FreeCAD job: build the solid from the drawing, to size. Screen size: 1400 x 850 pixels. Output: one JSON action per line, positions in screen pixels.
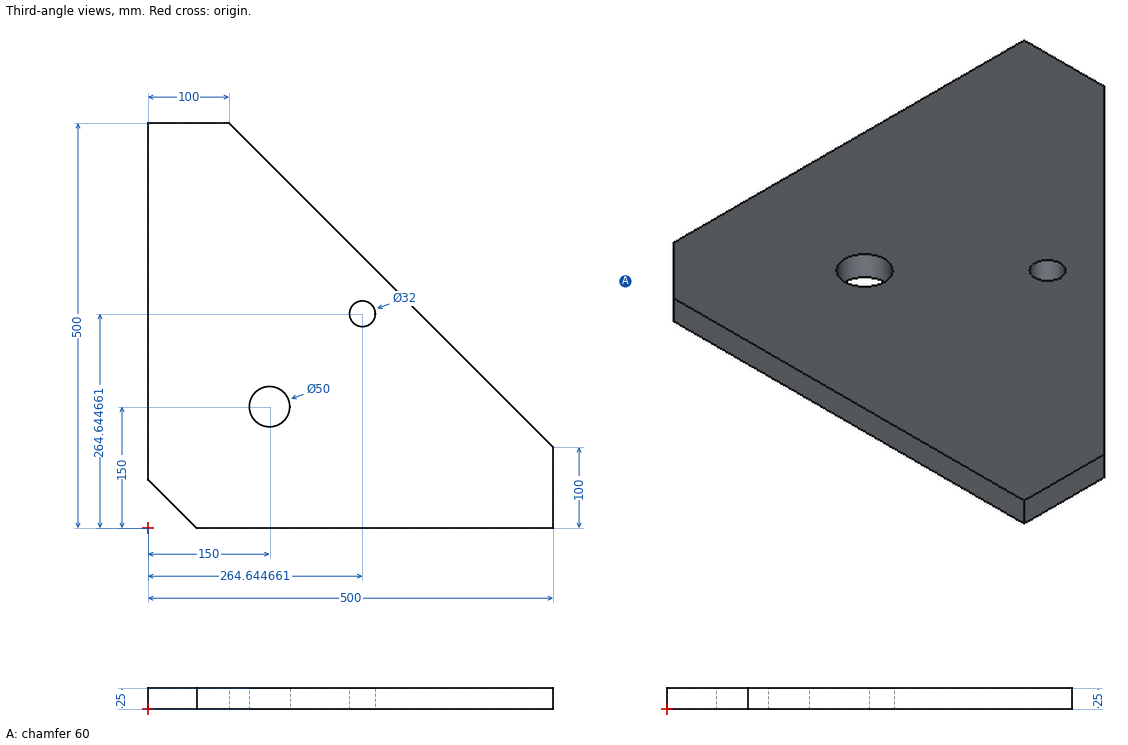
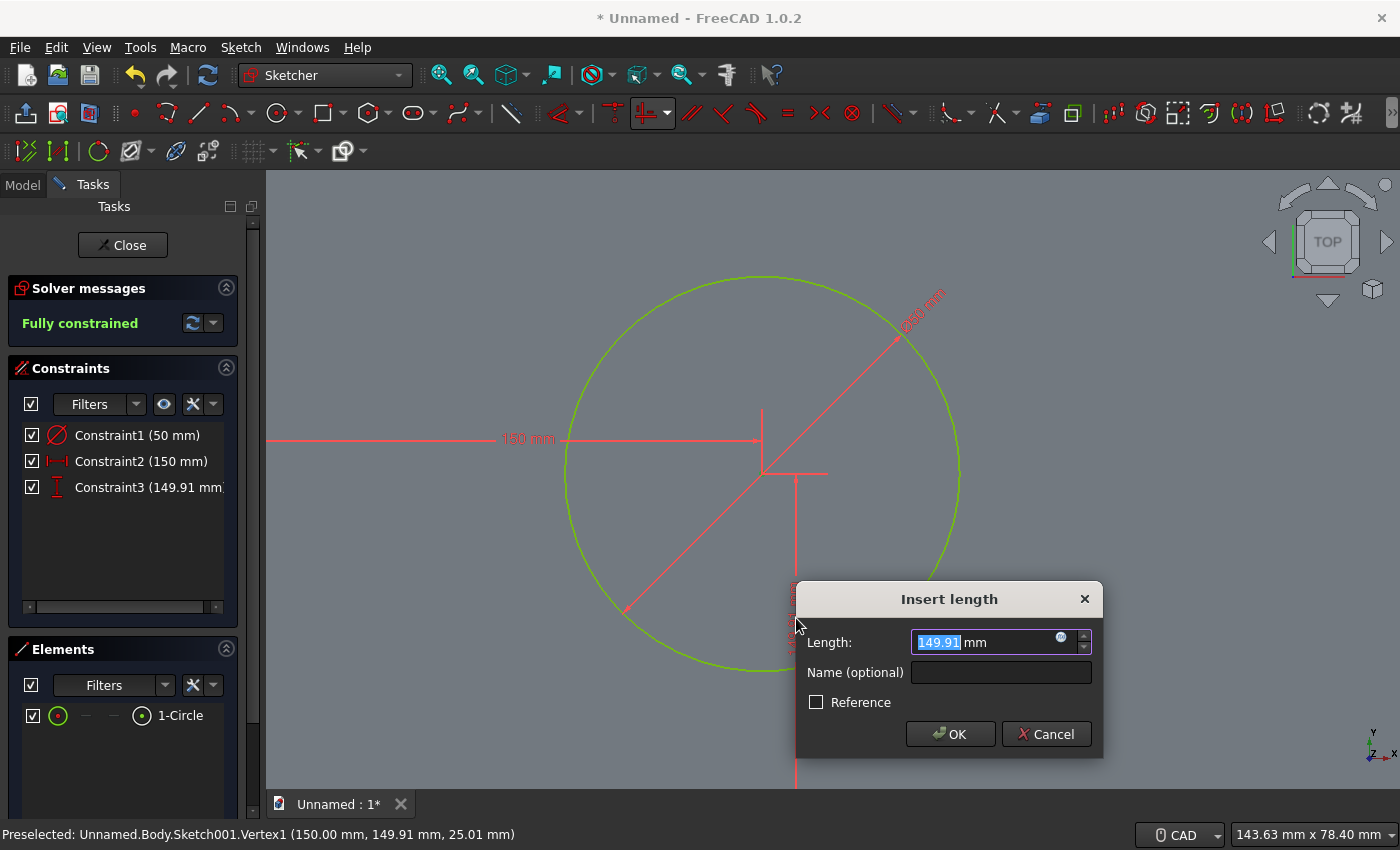
{"action": "type", "text": "150"}
{"action": "key", "text": "Return"}
{"action": "key", "text": "Escape"}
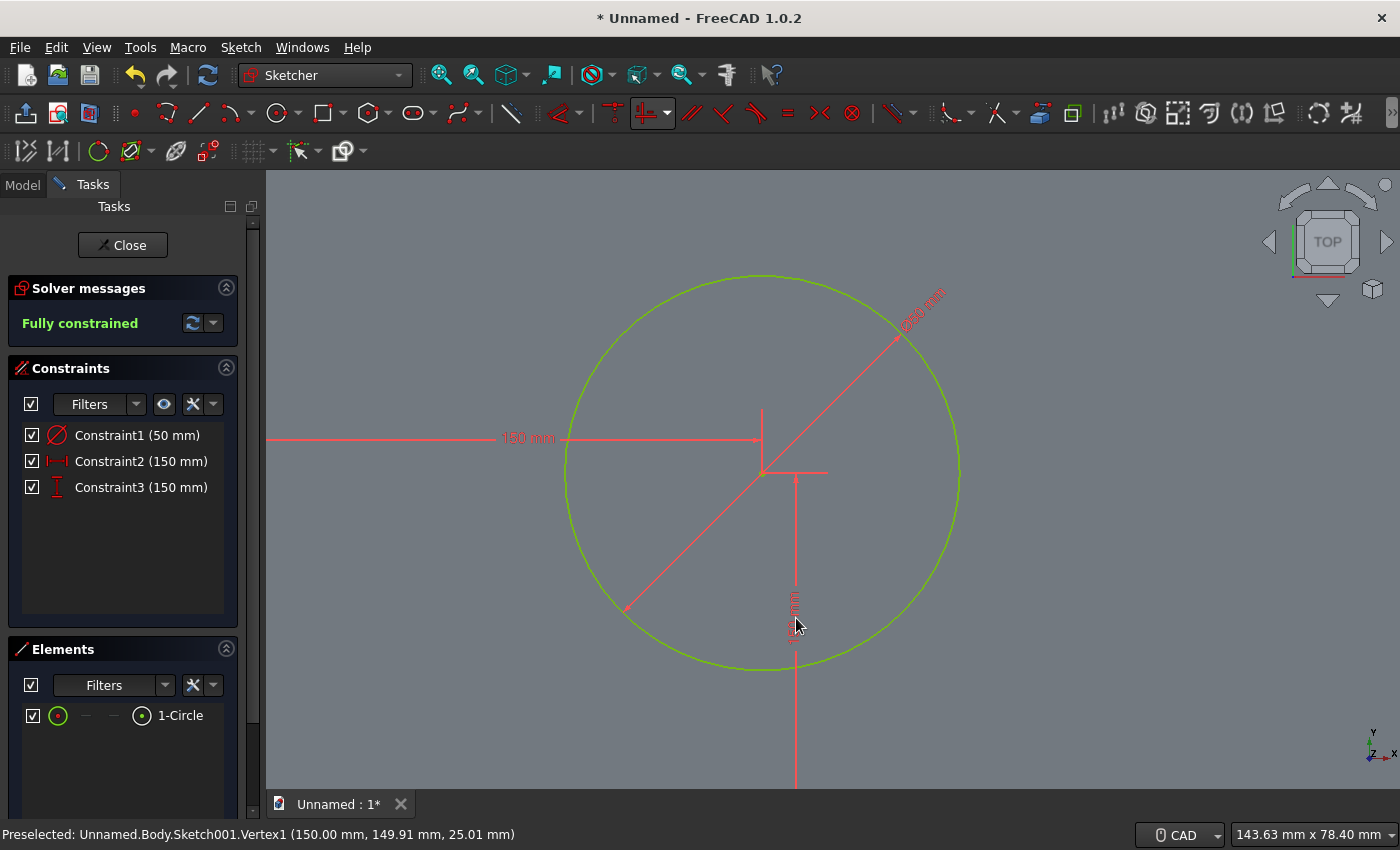
{"action": "left_click", "coordinate": [123, 245]}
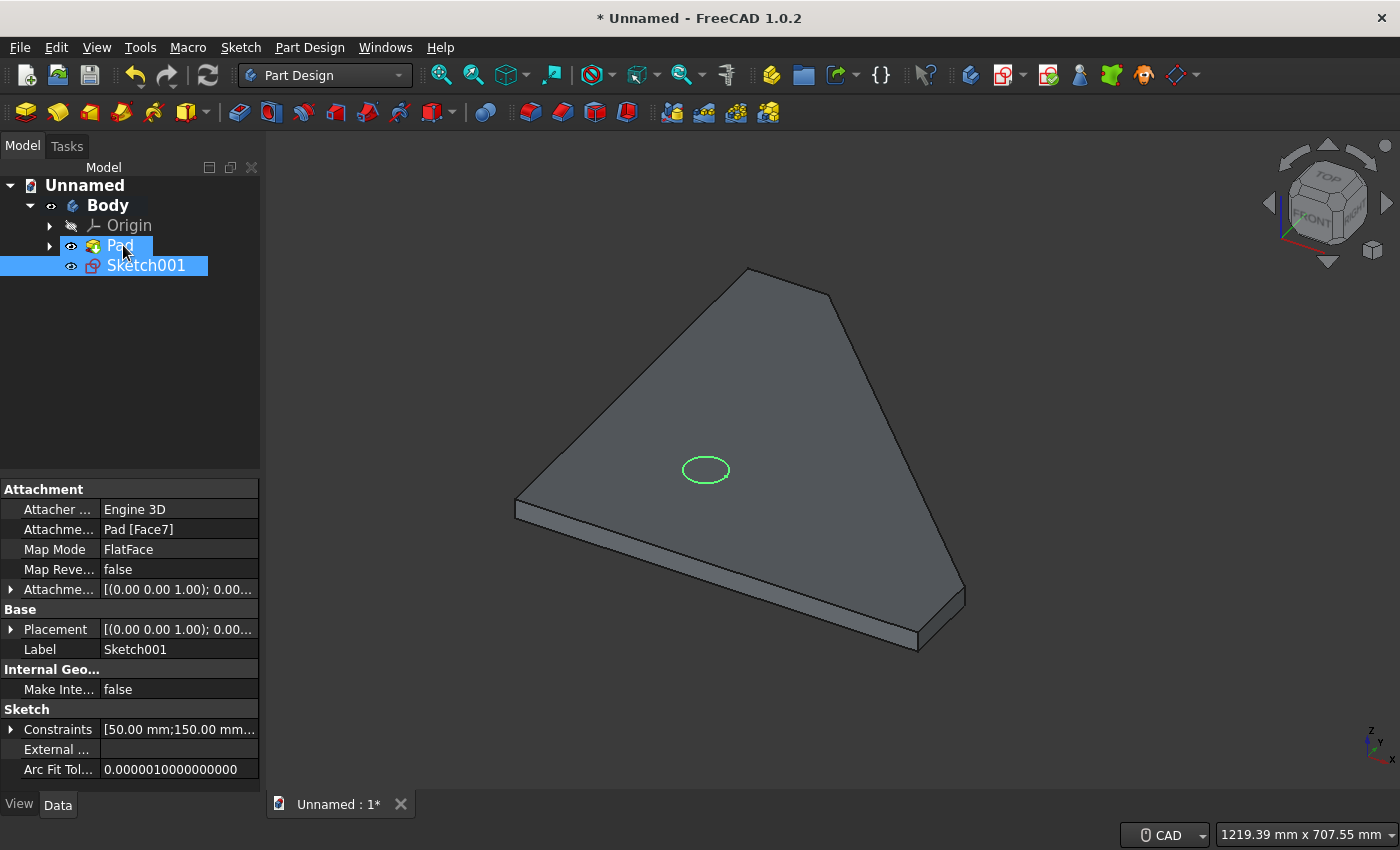
{"action": "left_click", "coordinate": [240, 112]}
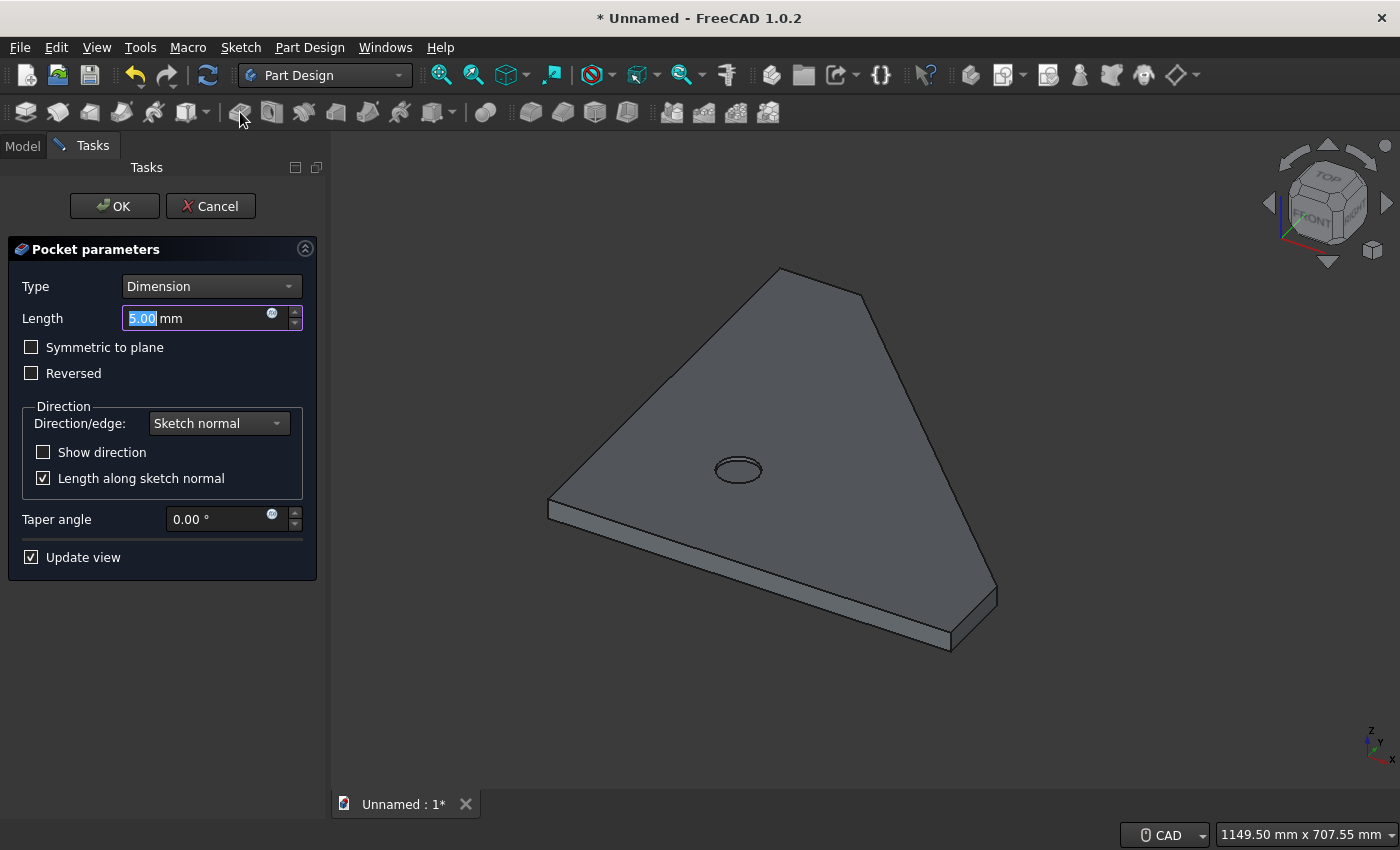
{"action": "type", "text": "25"}
{"action": "key", "text": "Tab"}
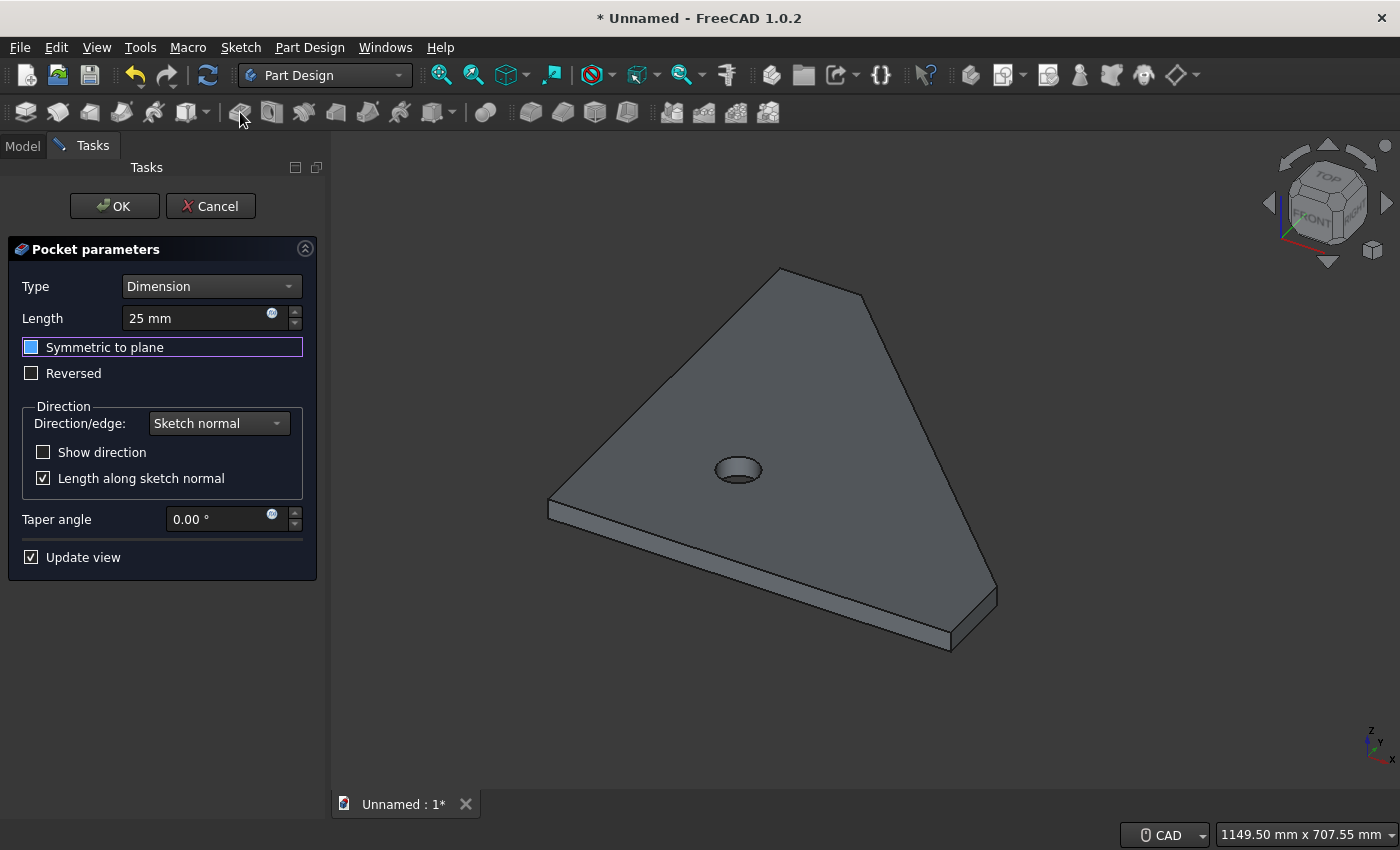
{"action": "left_click", "coordinate": [115, 206]}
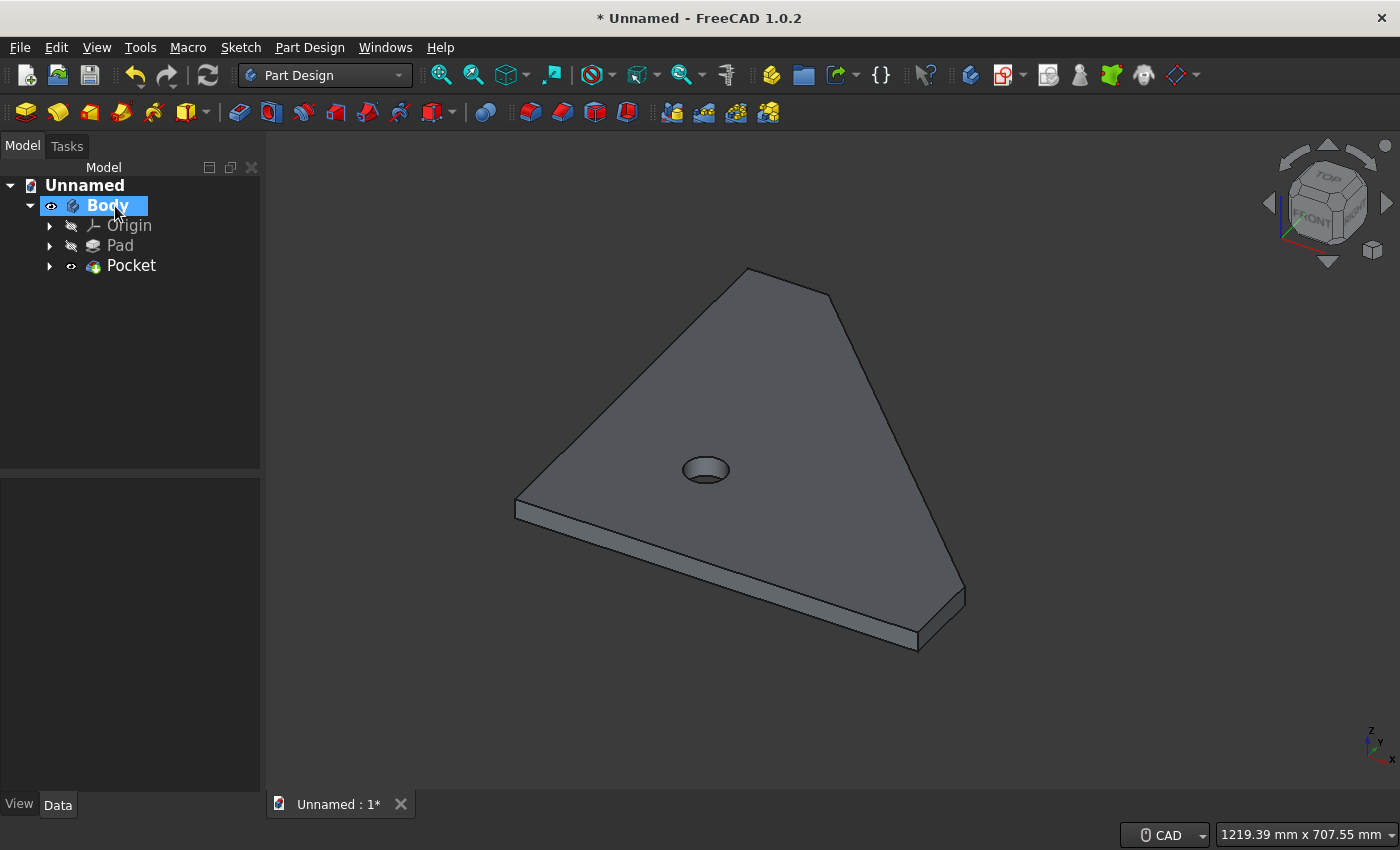
{"action": "key", "text": "0"}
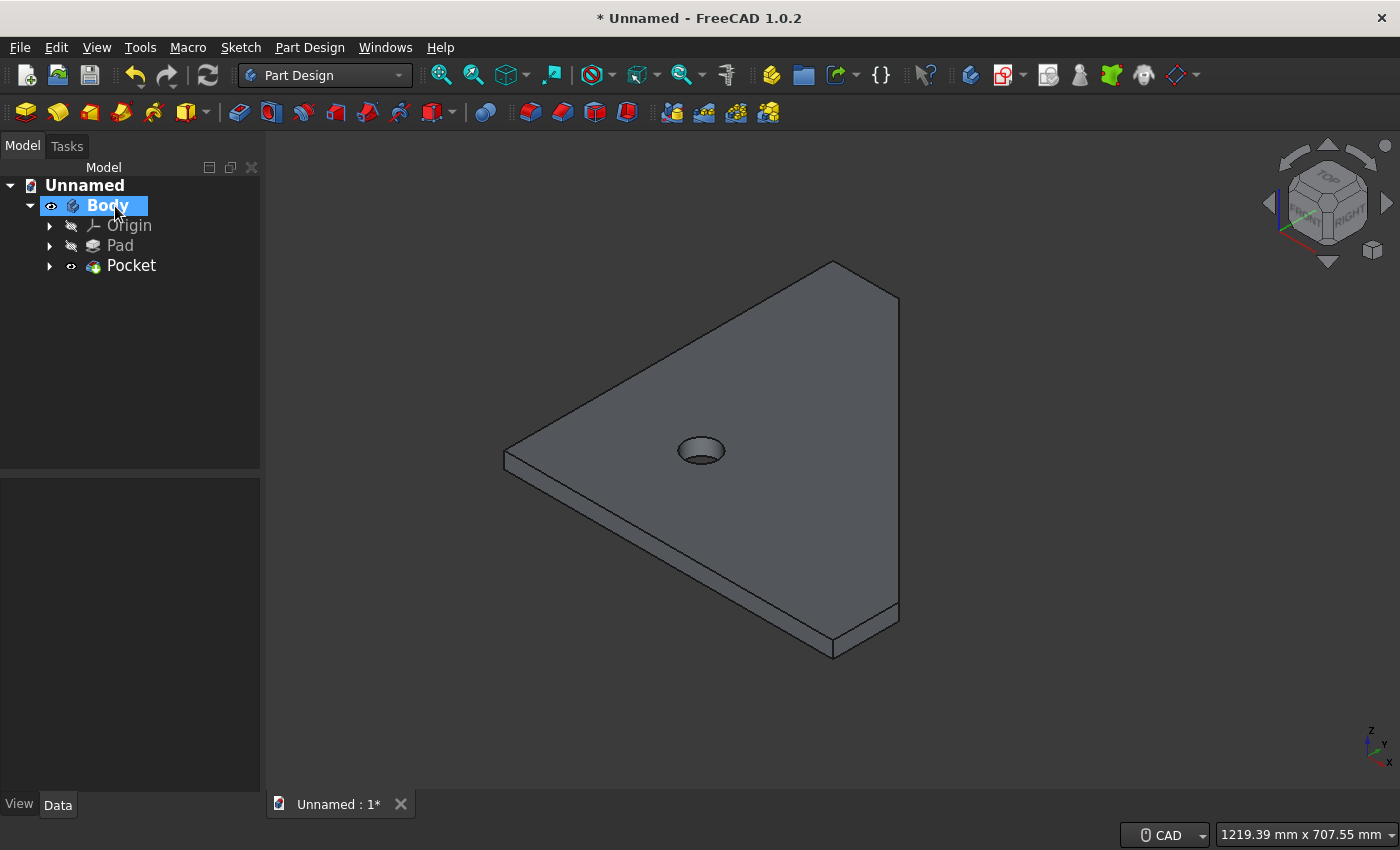
{"action": "key", "text": "2"}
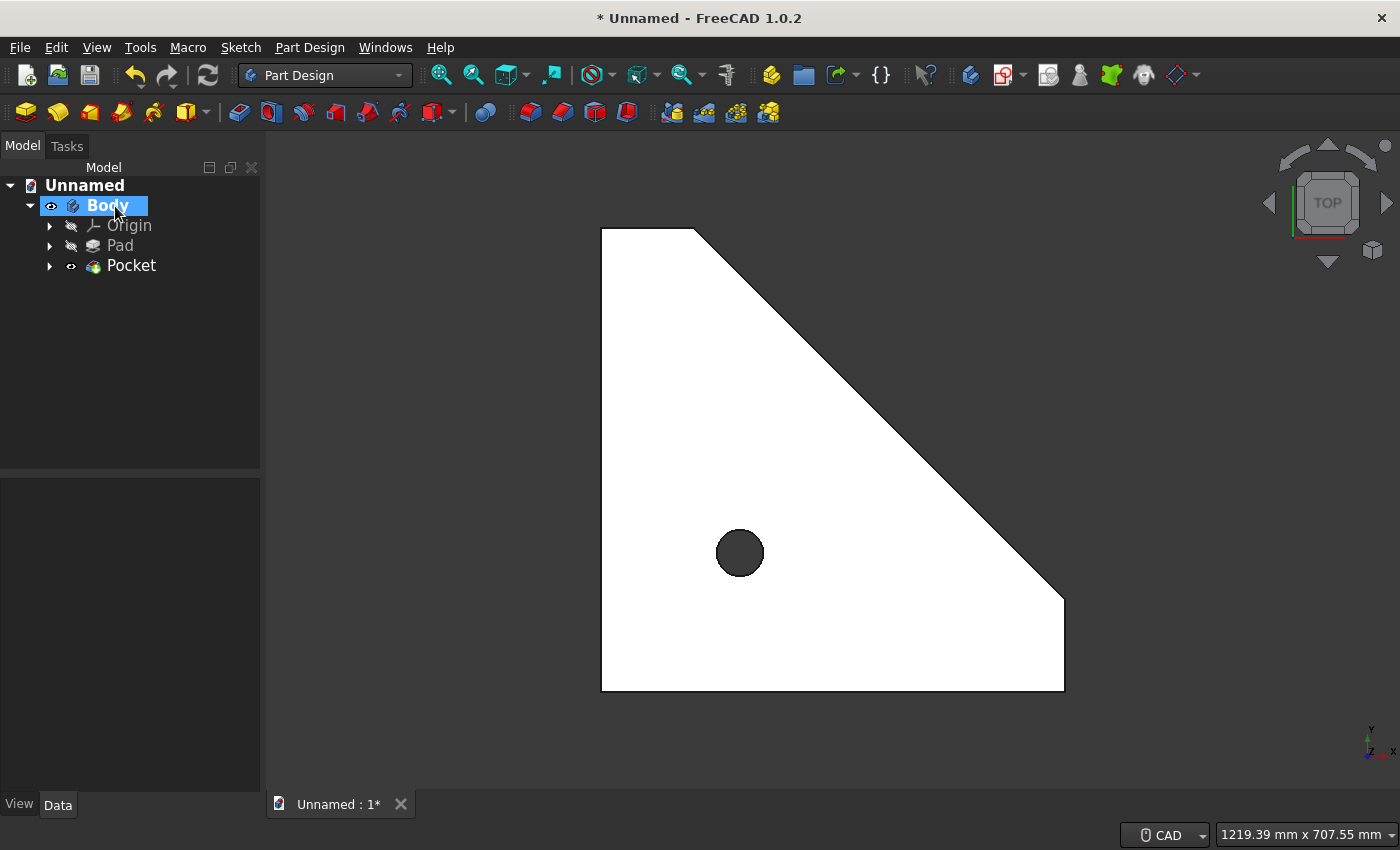
{"action": "key", "text": "1"}